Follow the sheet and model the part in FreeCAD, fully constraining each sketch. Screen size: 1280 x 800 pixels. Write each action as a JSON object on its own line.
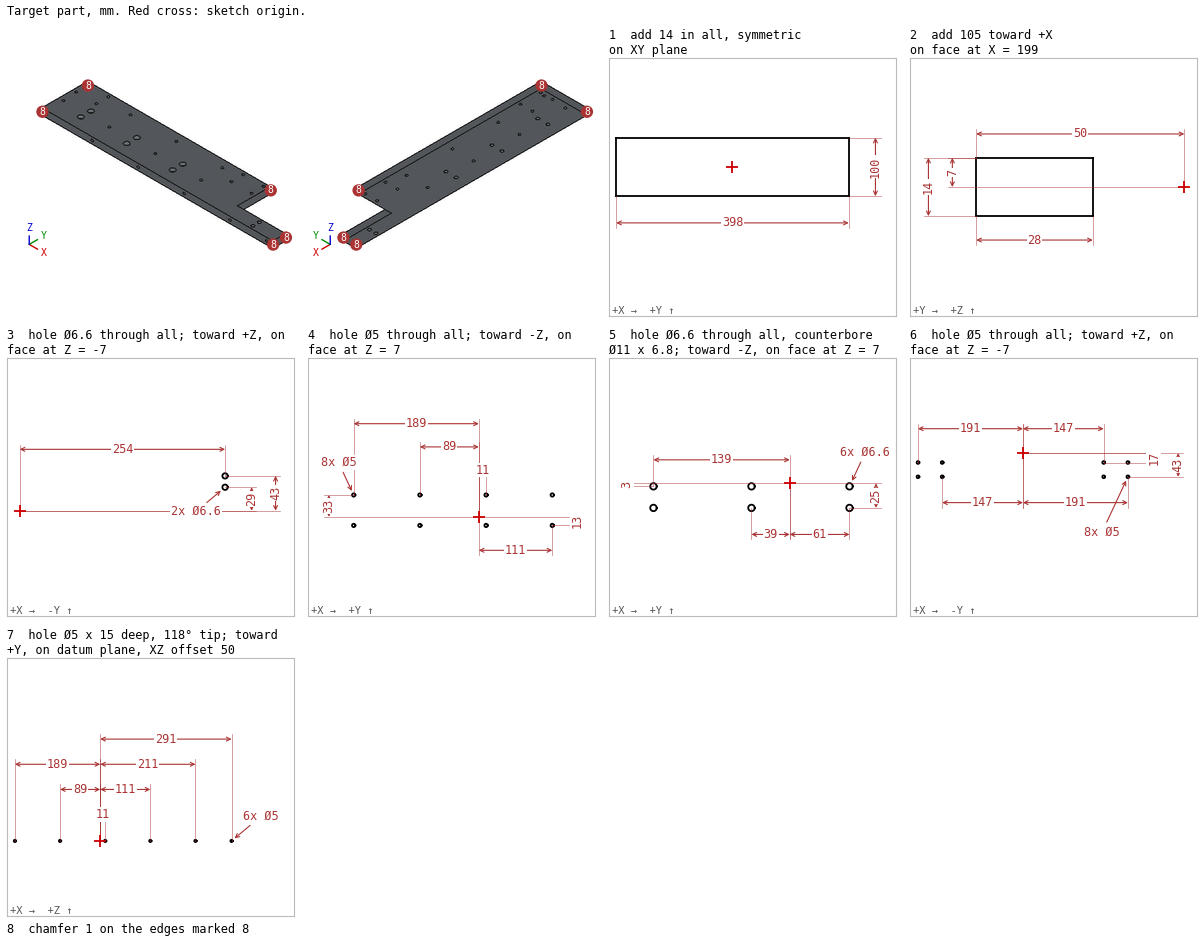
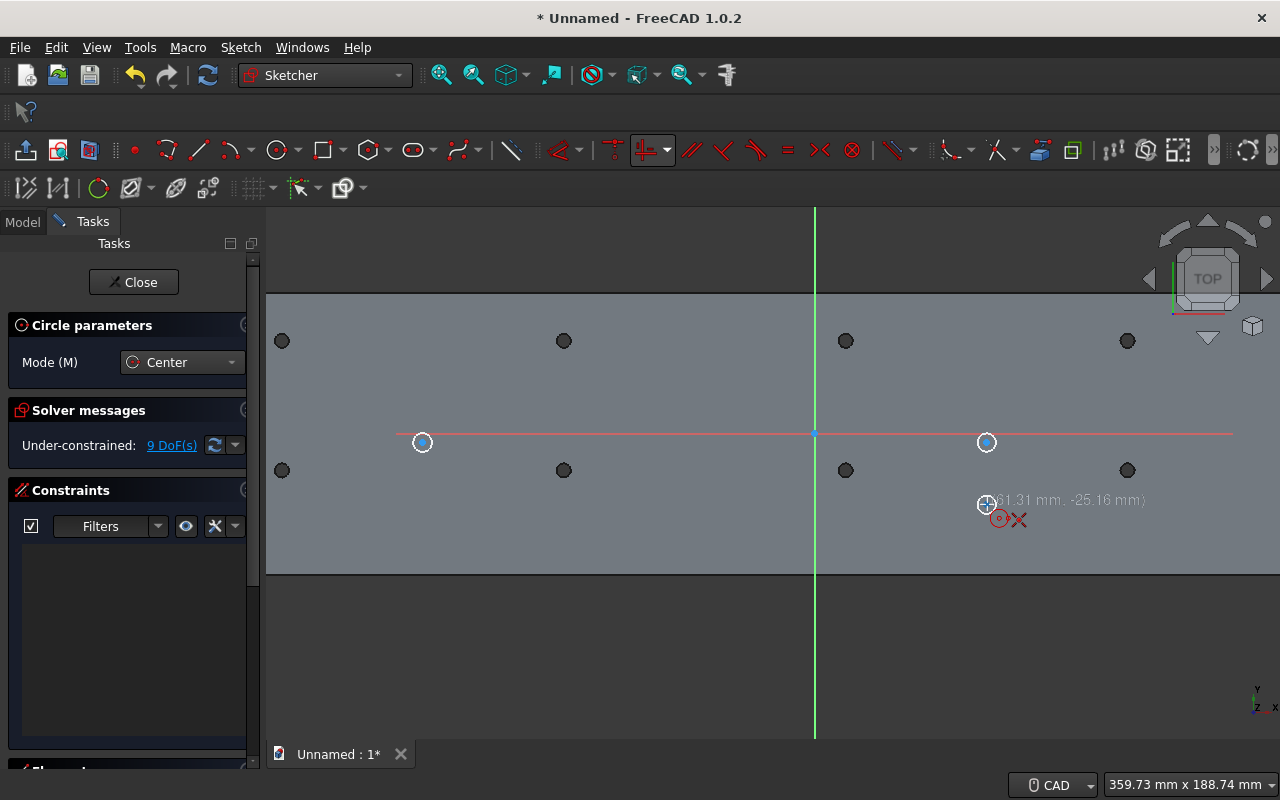
{"action": "scroll", "coordinate": [705, 504], "scroll_direction": "up", "scroll_amount": 5}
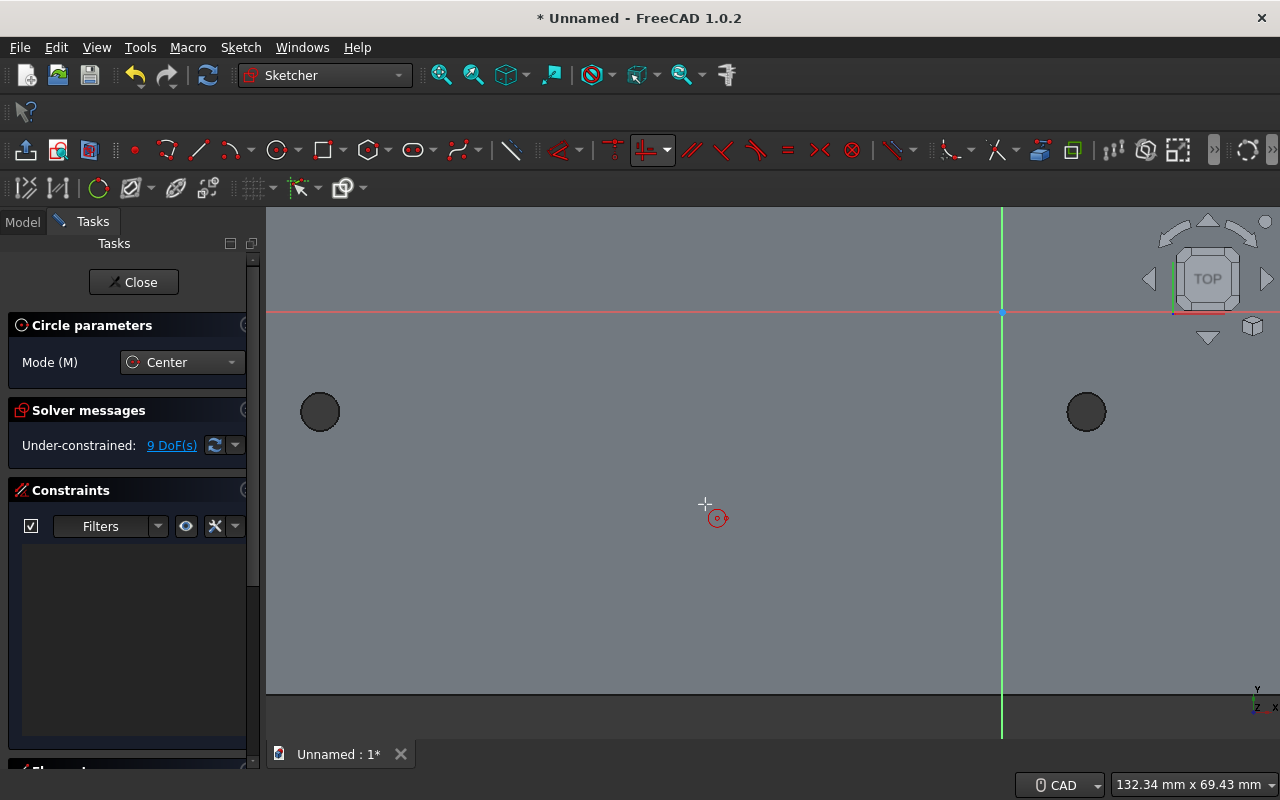
{"action": "left_click", "coordinate": [703, 504]}
{"action": "left_click", "coordinate": [721, 486]}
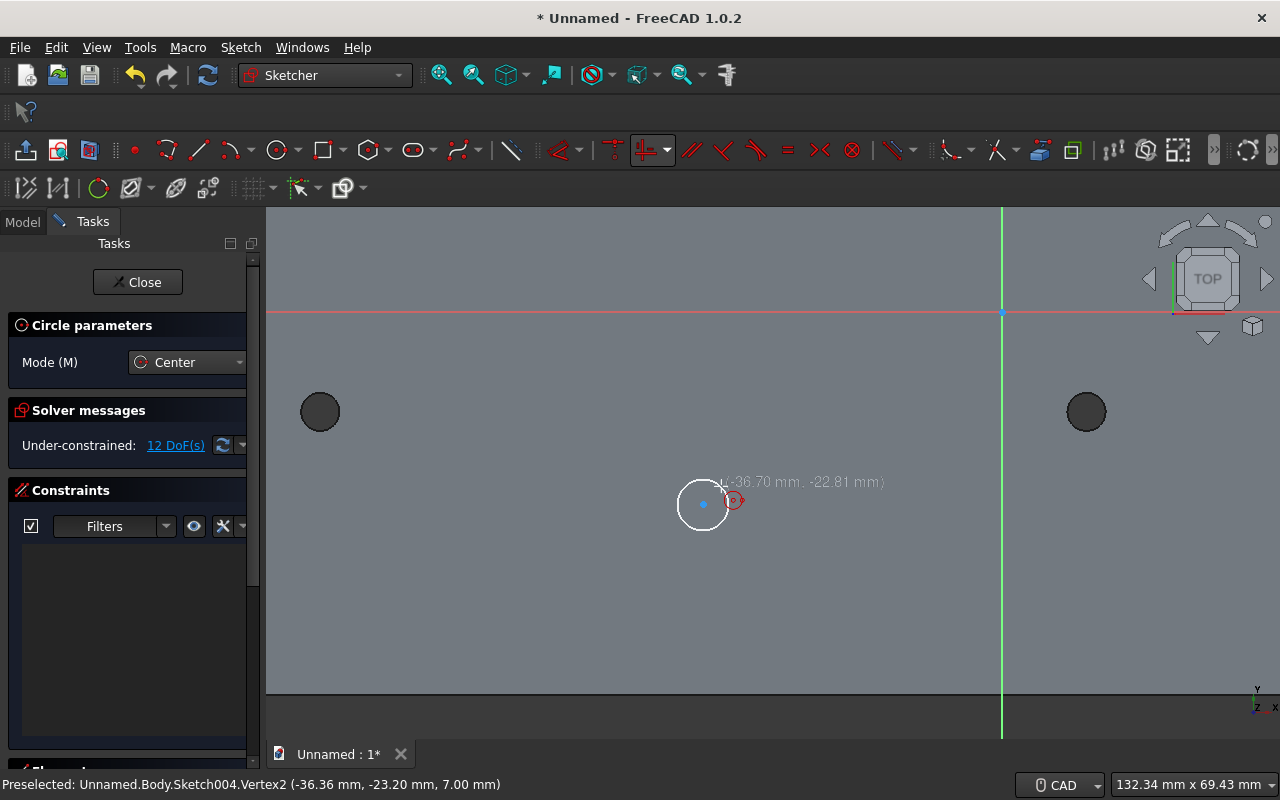
{"action": "left_click", "coordinate": [703, 335]}
{"action": "left_click", "coordinate": [721, 353]}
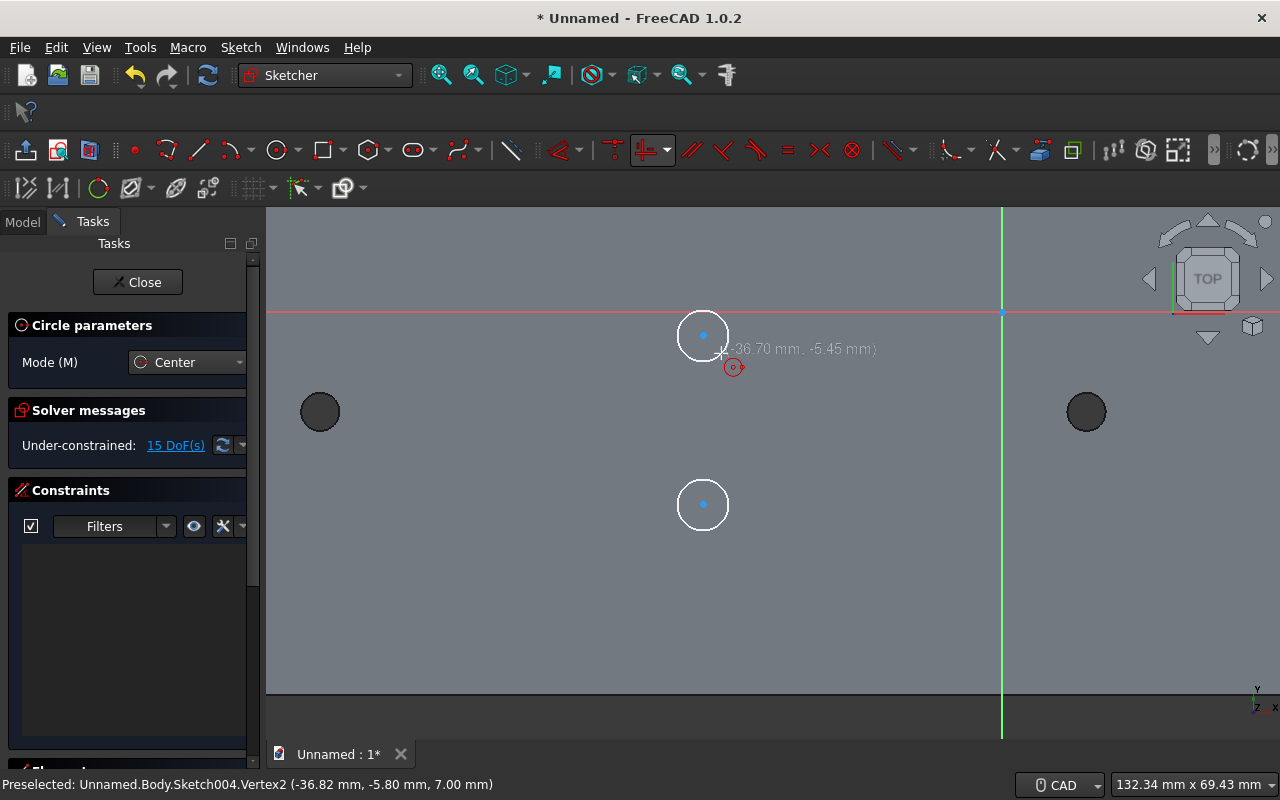
{"action": "scroll", "coordinate": [705, 504], "scroll_direction": "down", "scroll_amount": 5}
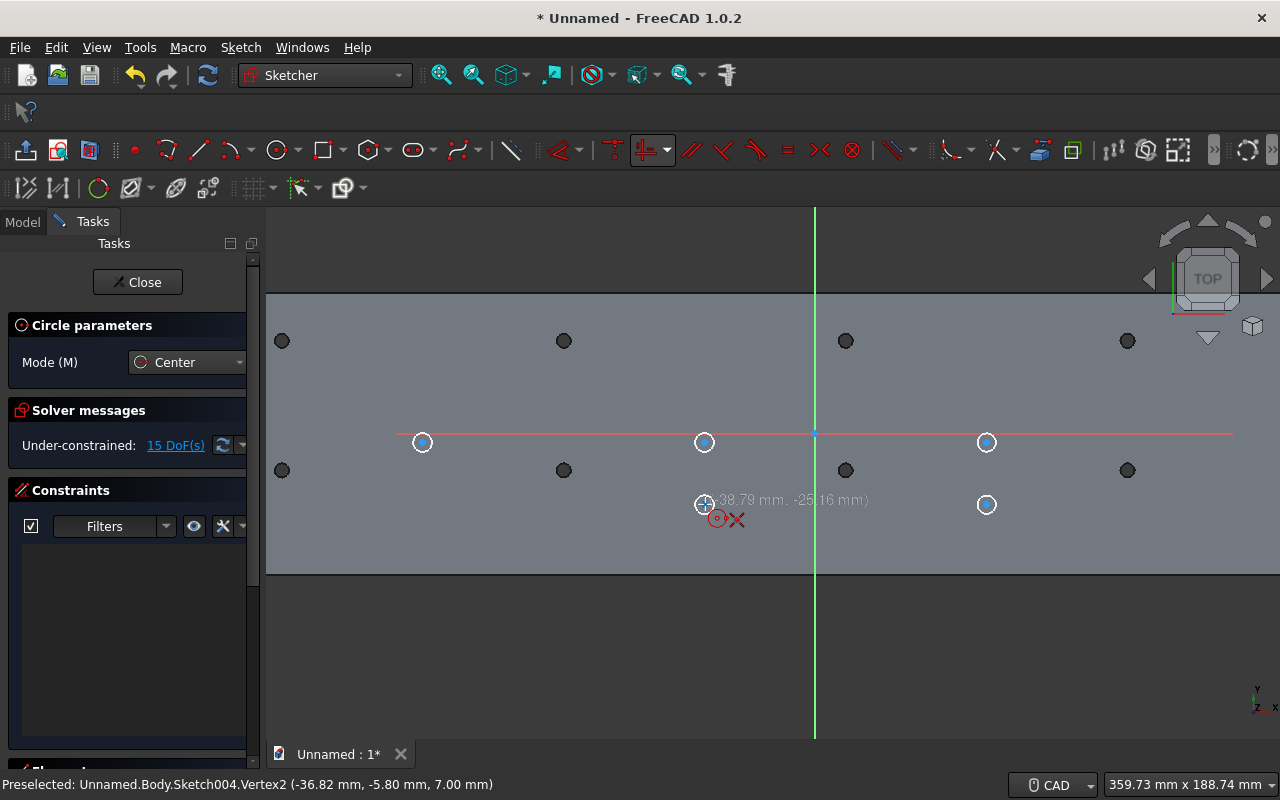
{"action": "scroll", "coordinate": [423, 504], "scroll_direction": "up", "scroll_amount": 5}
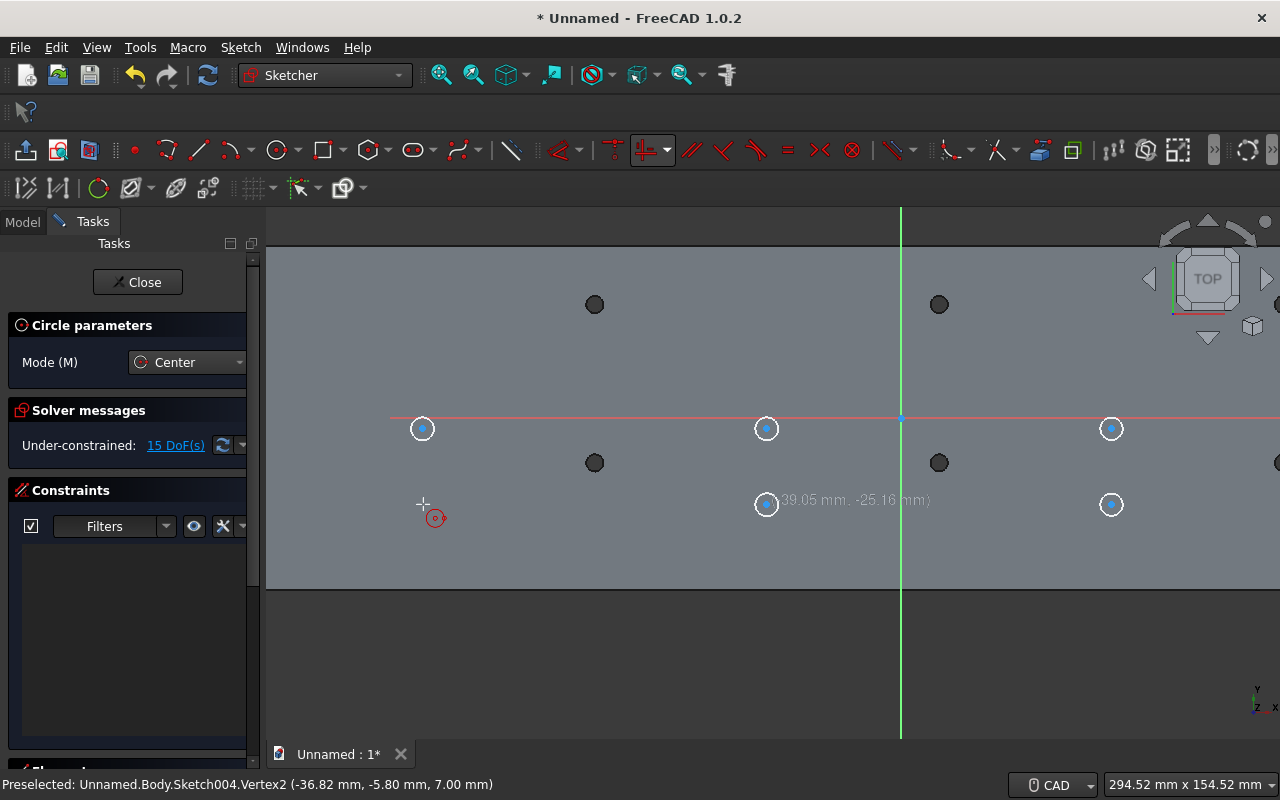
{"action": "left_click", "coordinate": [422, 504]}
{"action": "left_click", "coordinate": [440, 486]}
{"action": "key", "text": "Escape"}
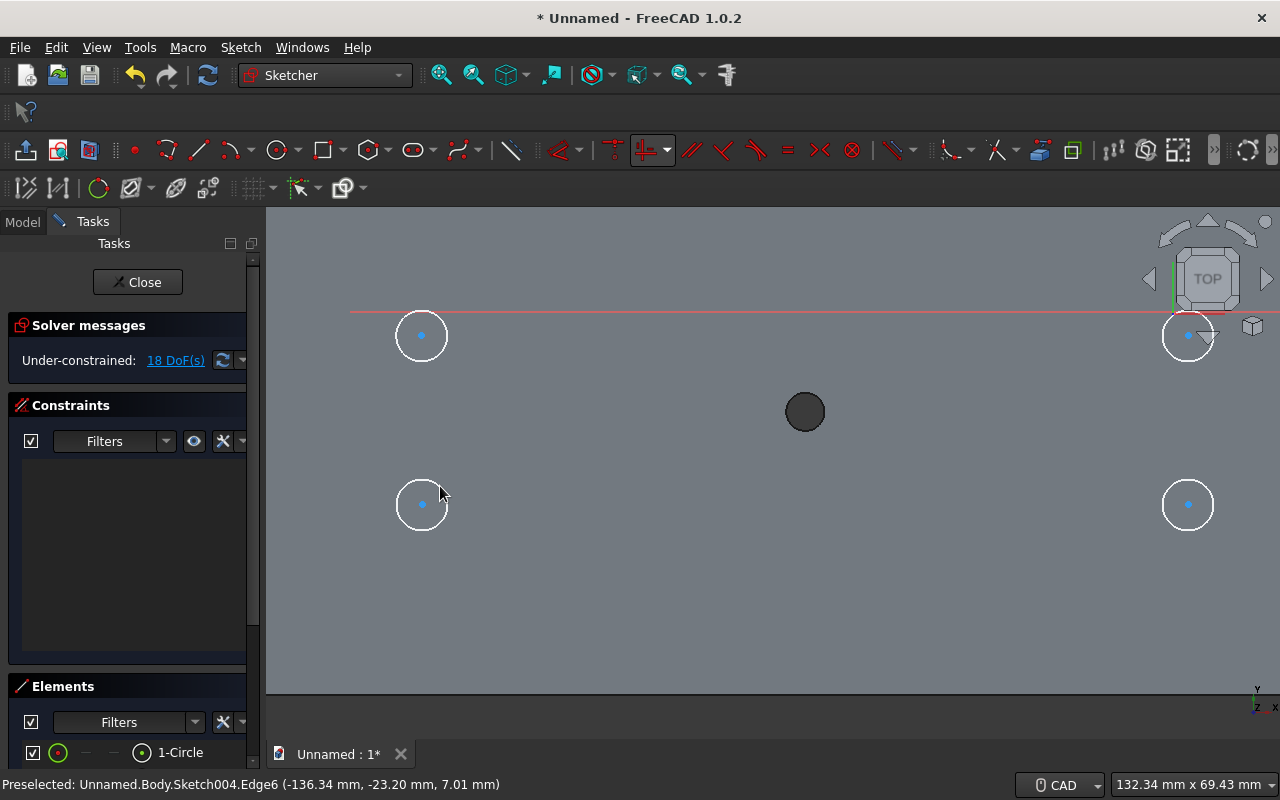
{"action": "left_click", "coordinate": [404, 354]}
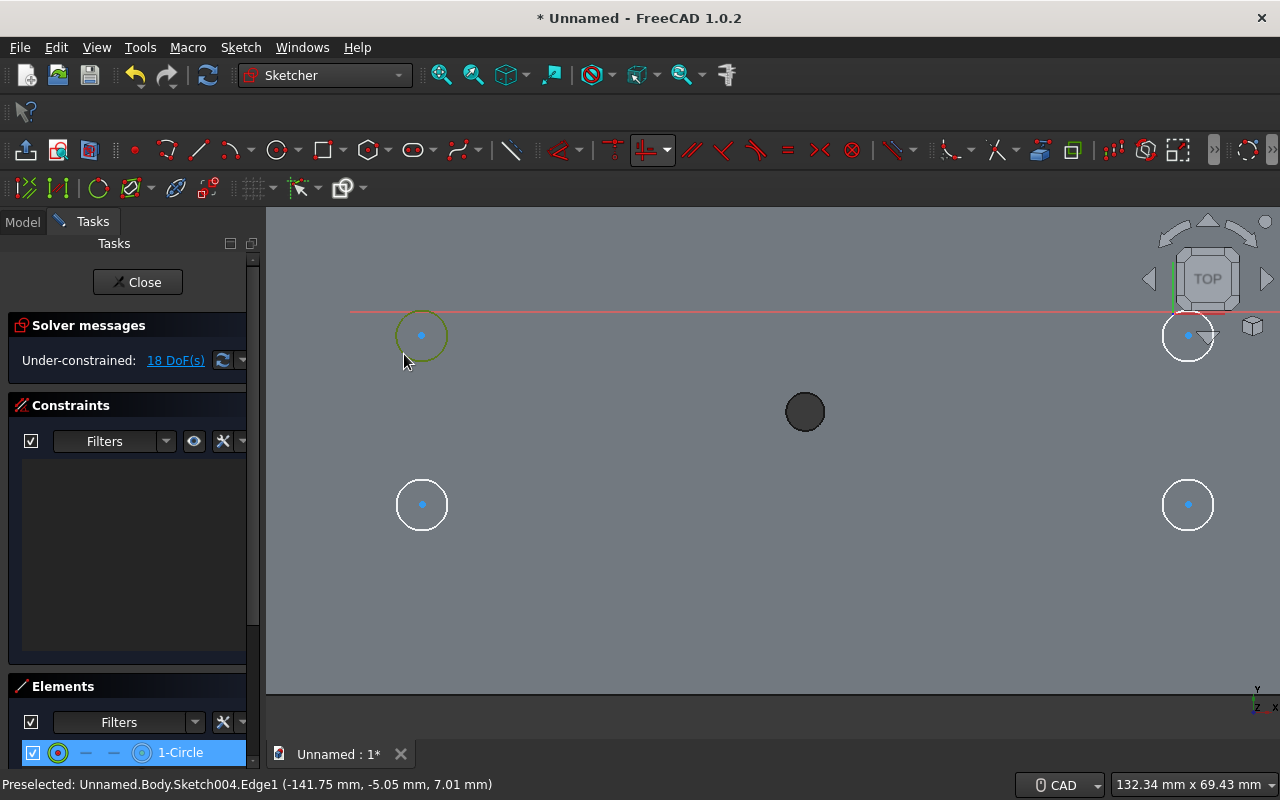
{"action": "scroll", "coordinate": [423, 504], "scroll_direction": "down", "scroll_amount": 5}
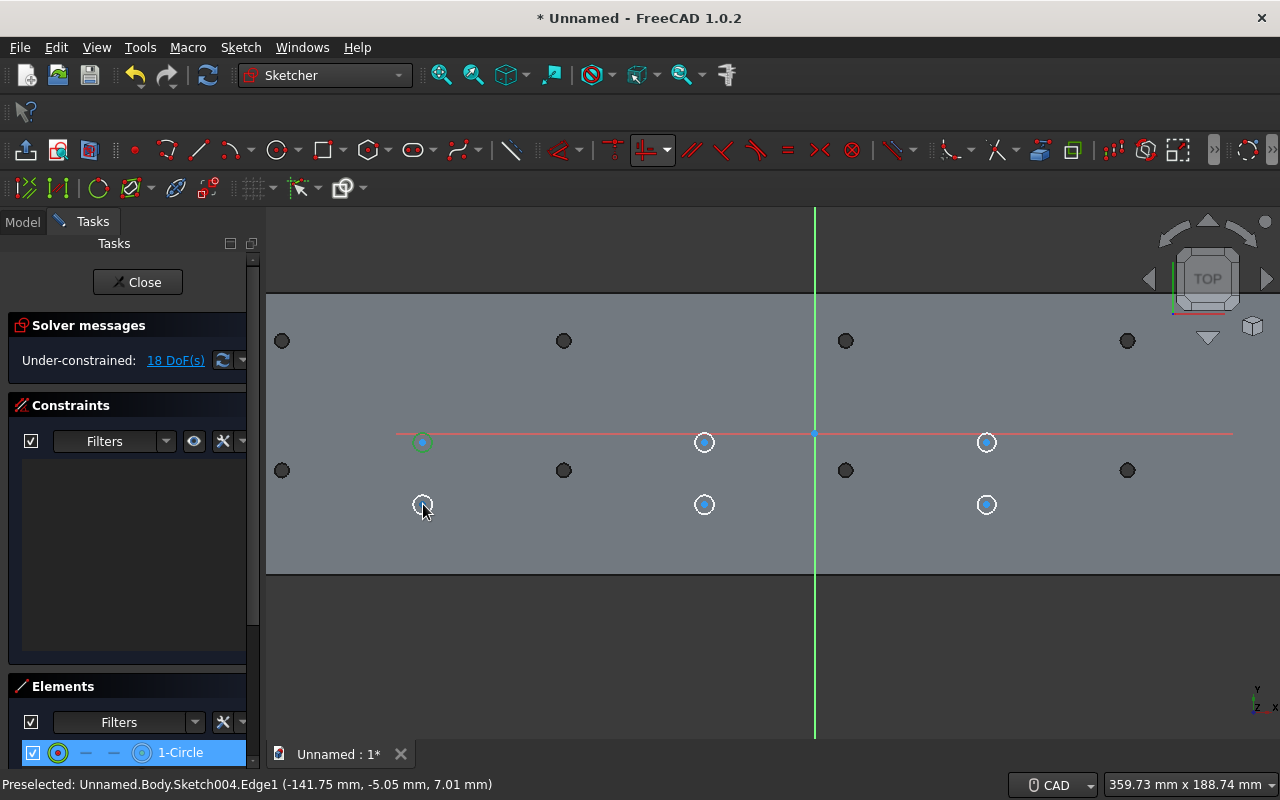
{"action": "scroll", "coordinate": [993, 498], "scroll_direction": "up", "scroll_amount": 3}